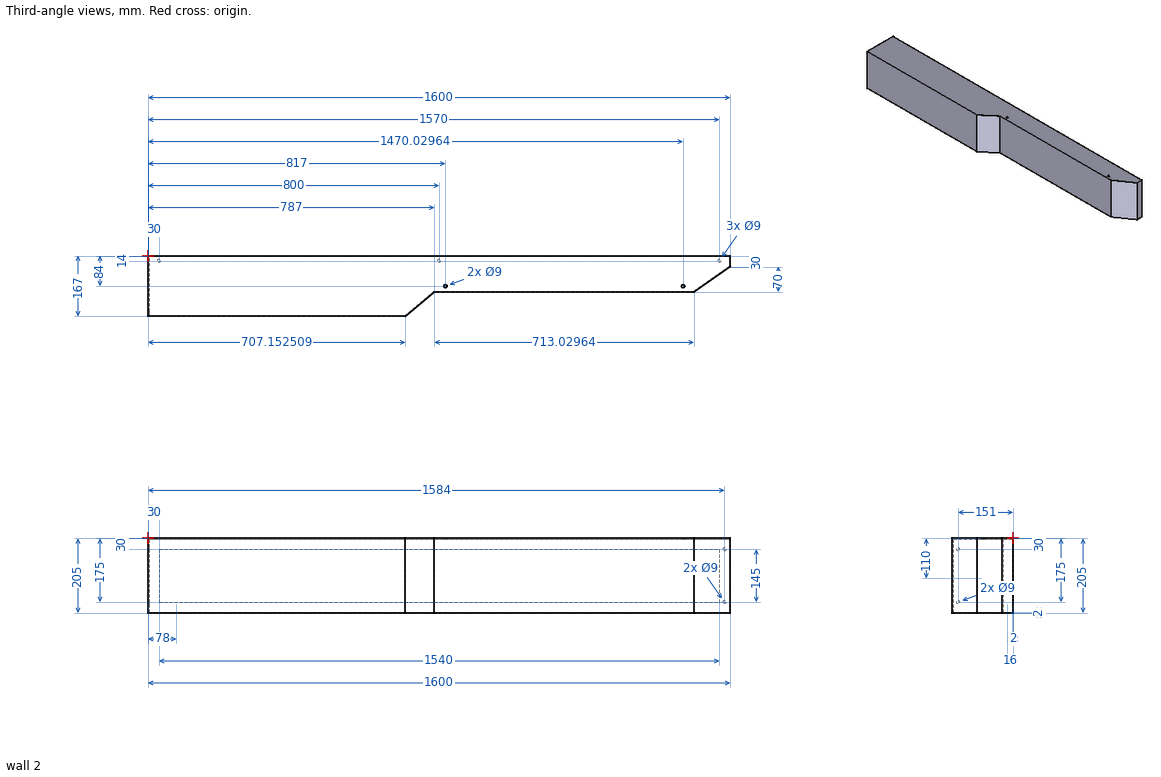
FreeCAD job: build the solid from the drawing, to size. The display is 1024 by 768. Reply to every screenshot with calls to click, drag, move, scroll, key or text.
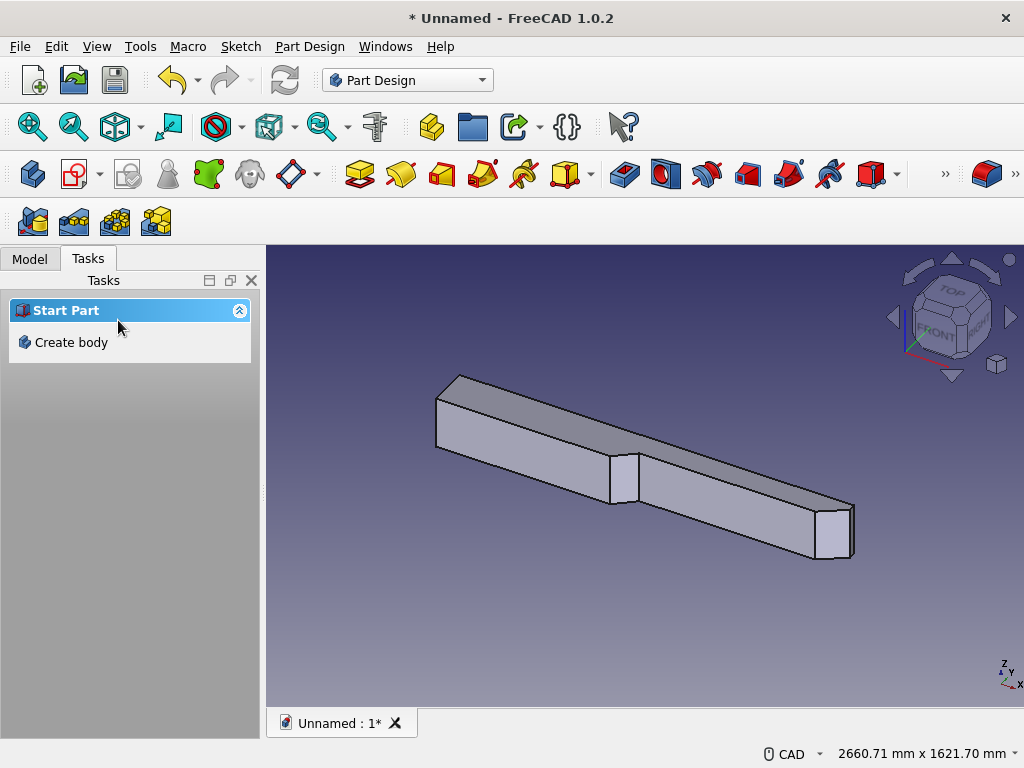
key(0)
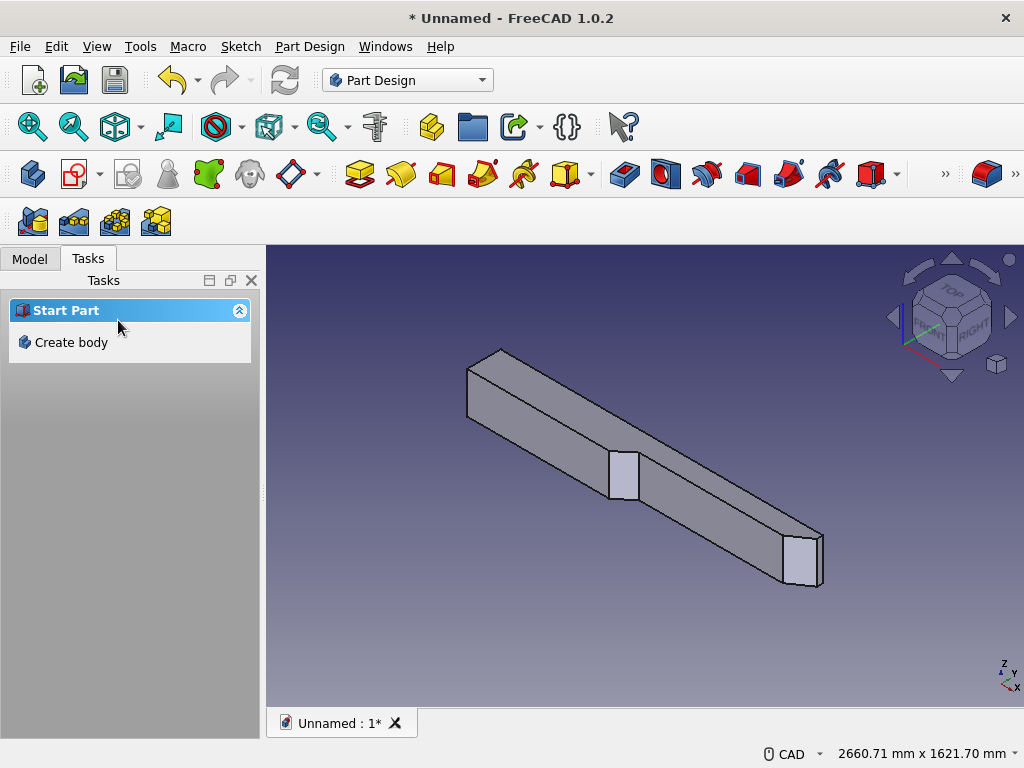
key(2)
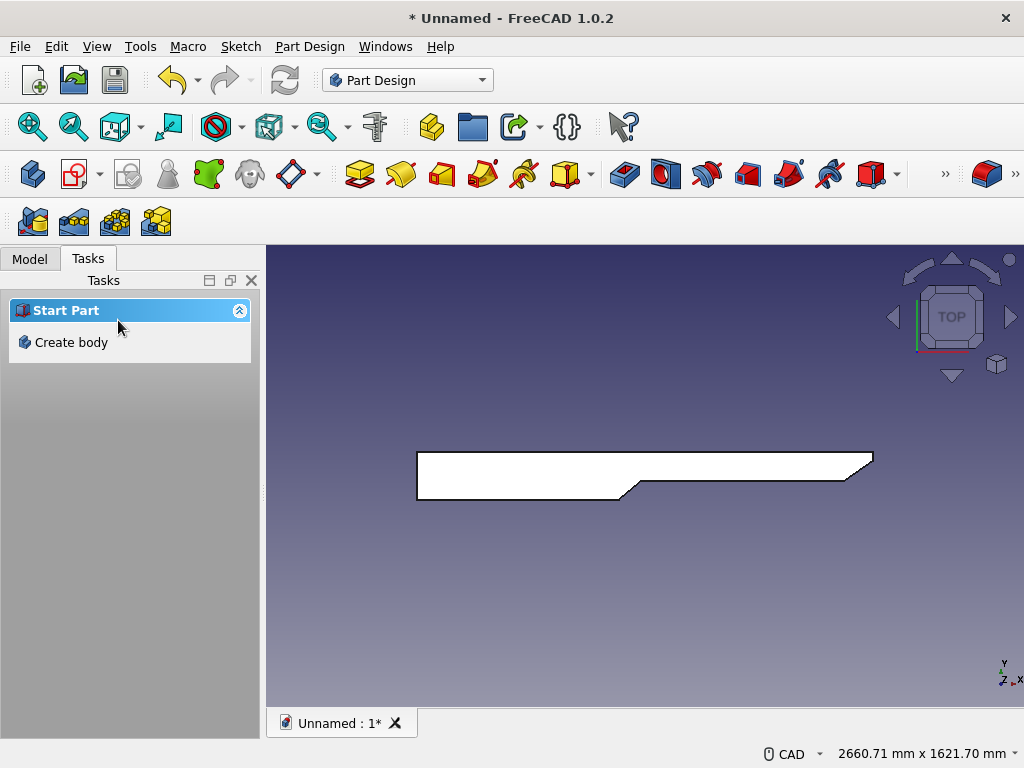
key(1)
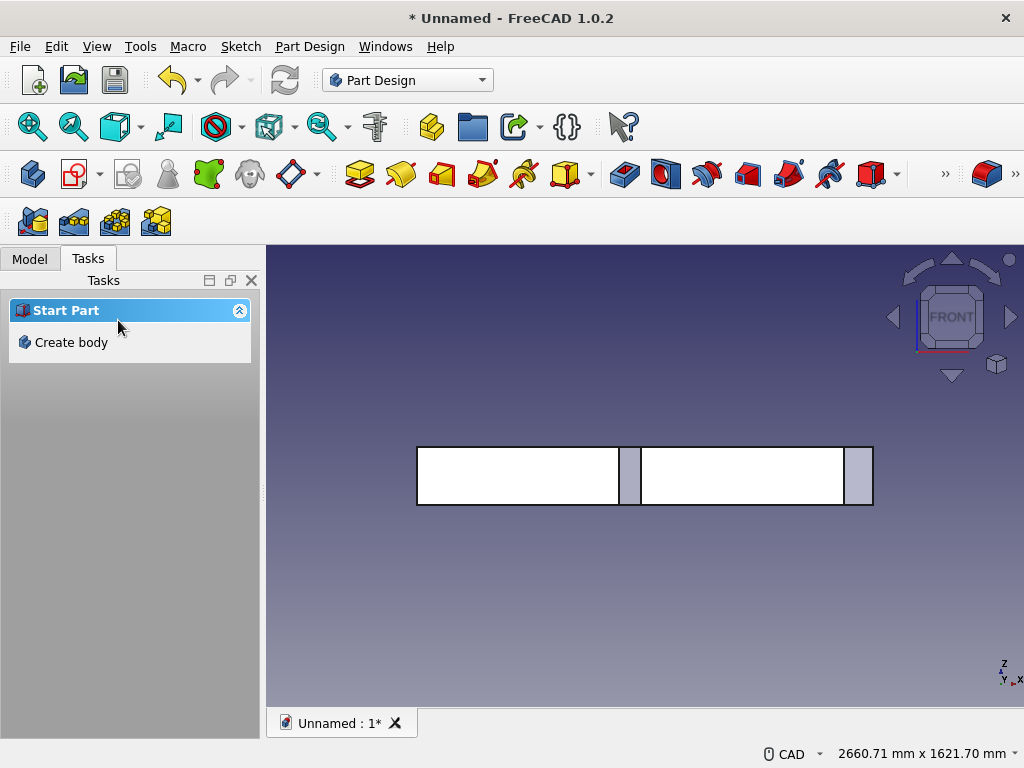
key(3)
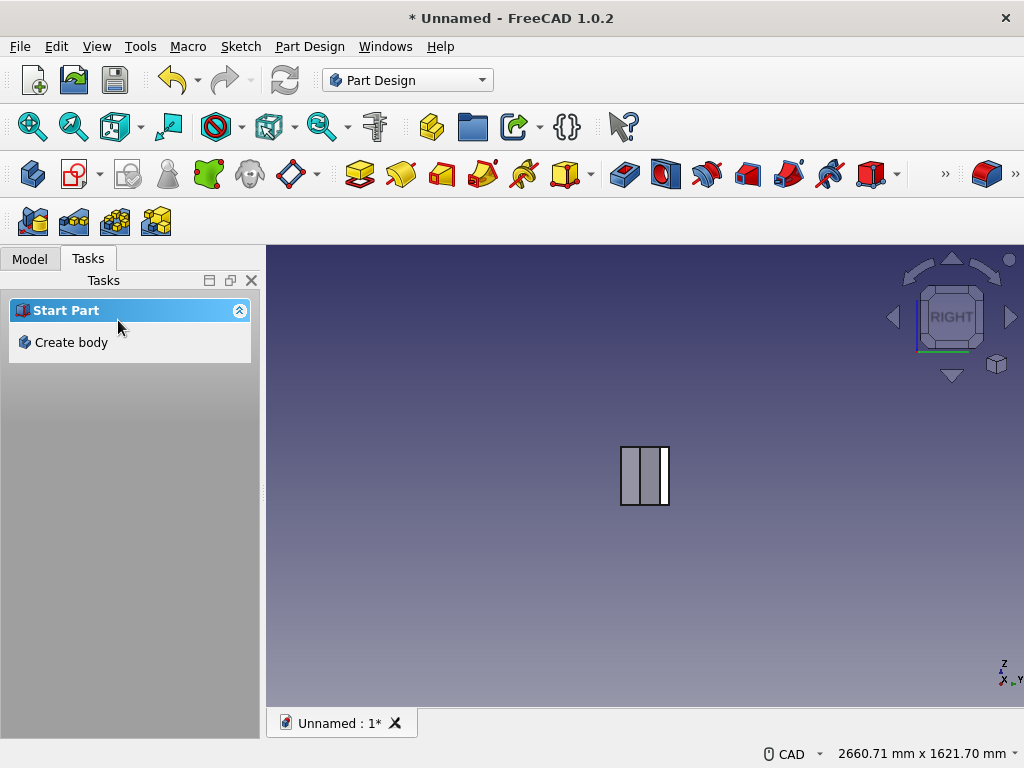
key(v)
key(f)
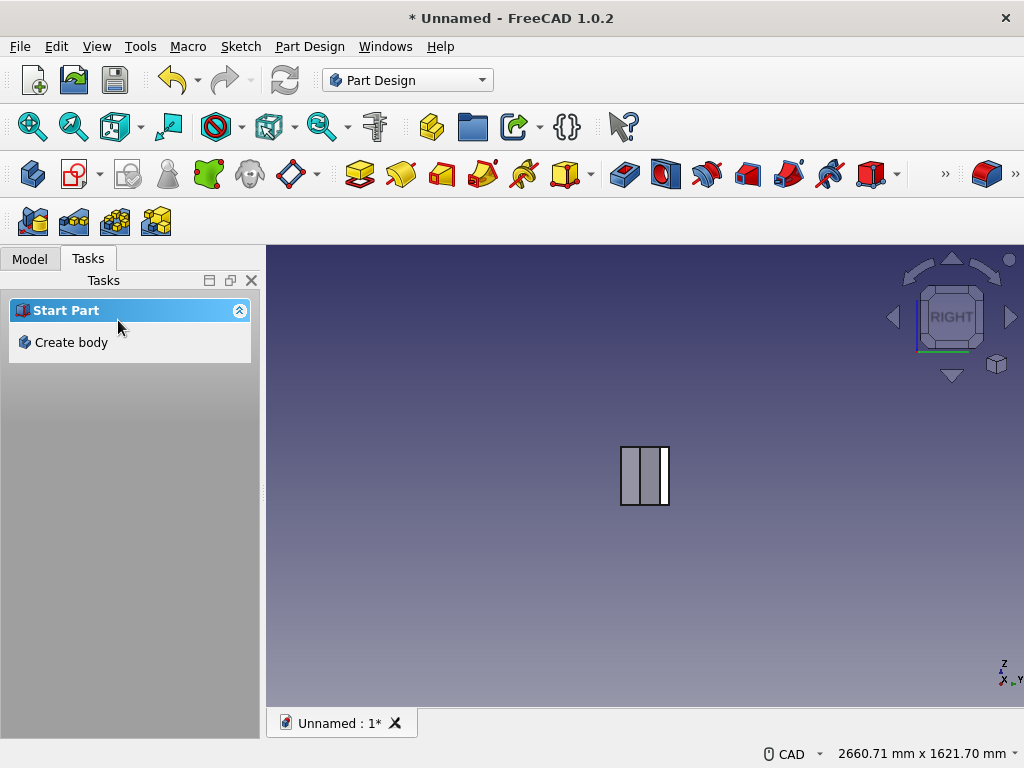
key(5)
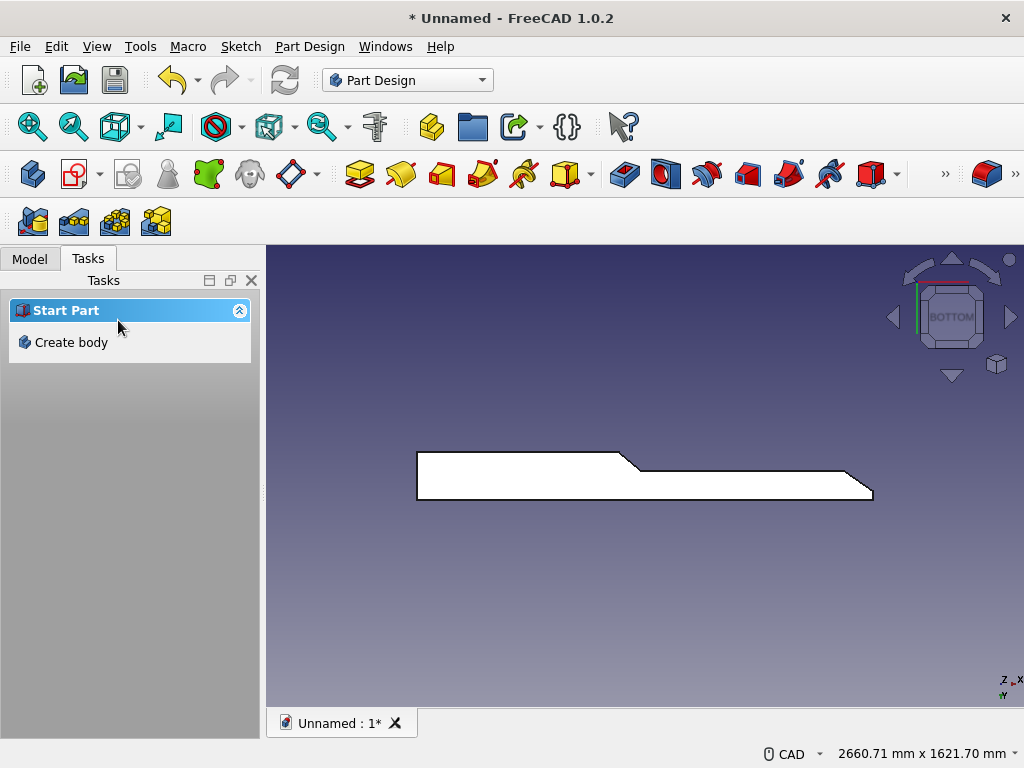
key(4)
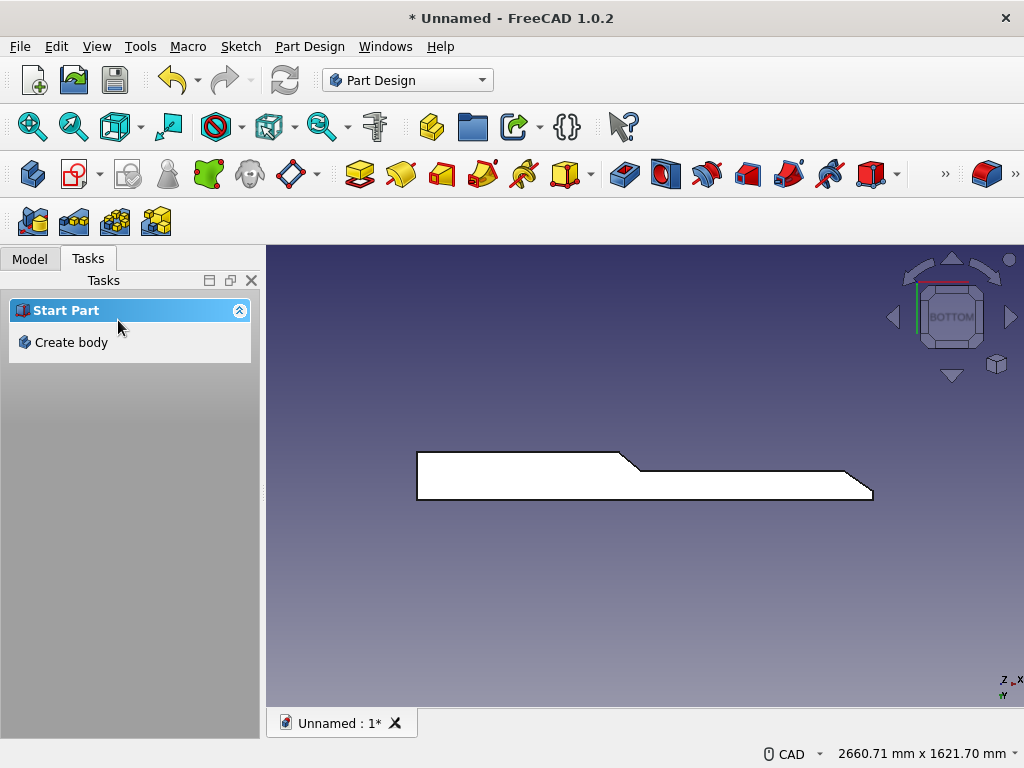
click(450, 475)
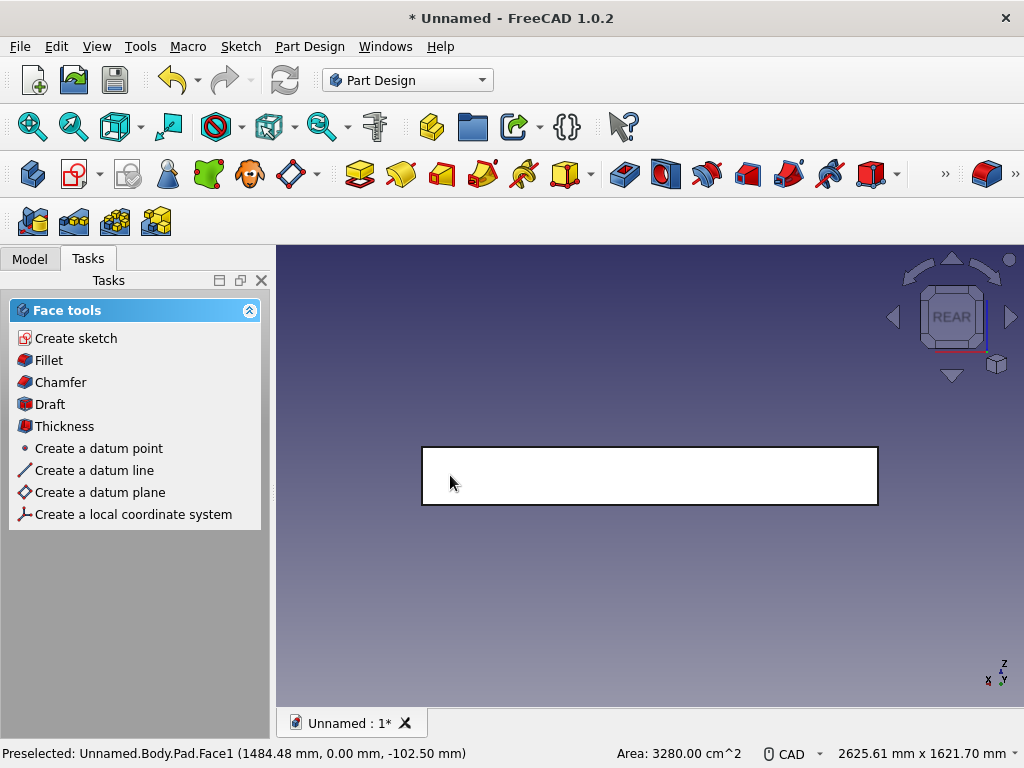
click(135, 426)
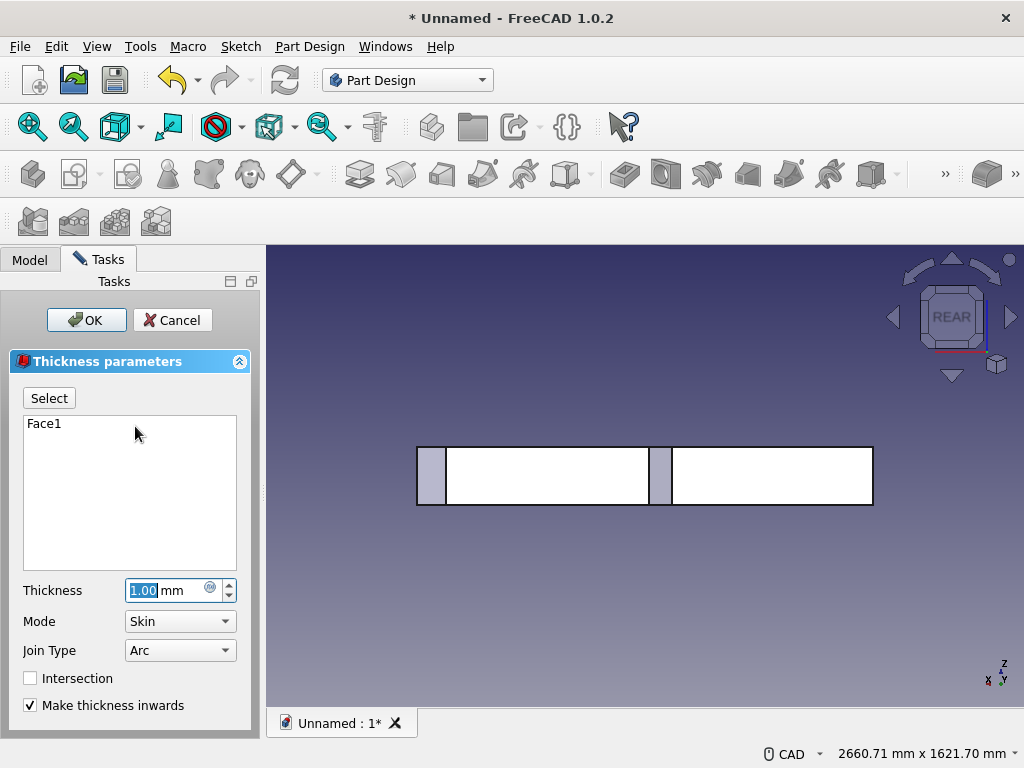
text(2)
key(Tab)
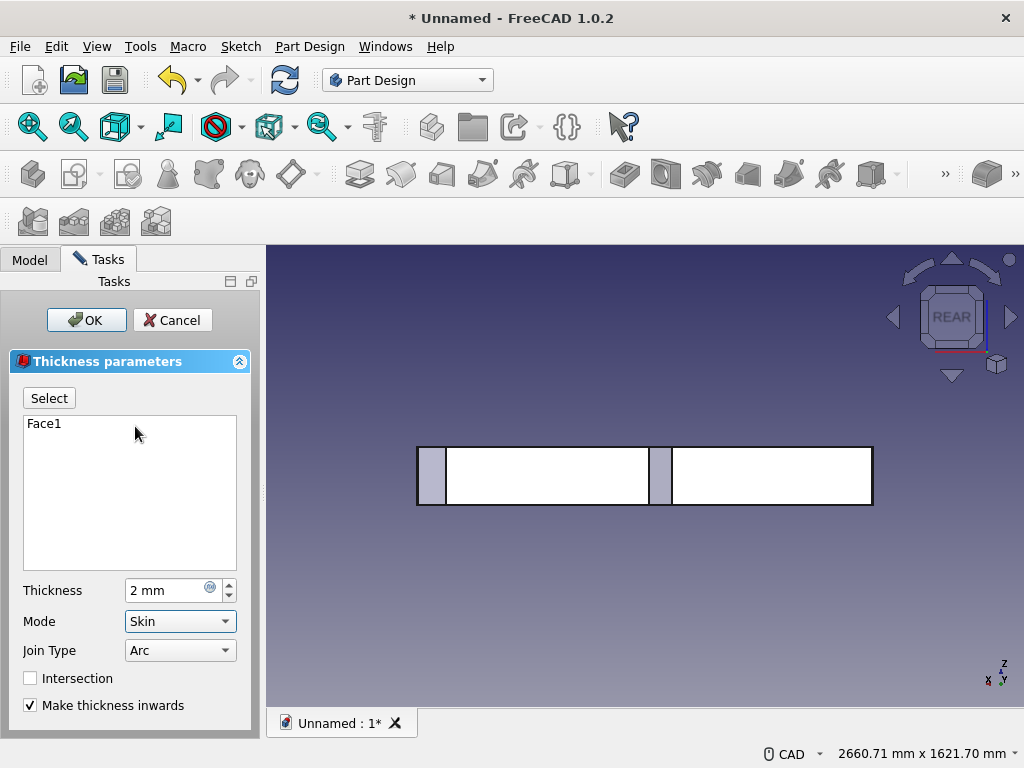
click(181, 650)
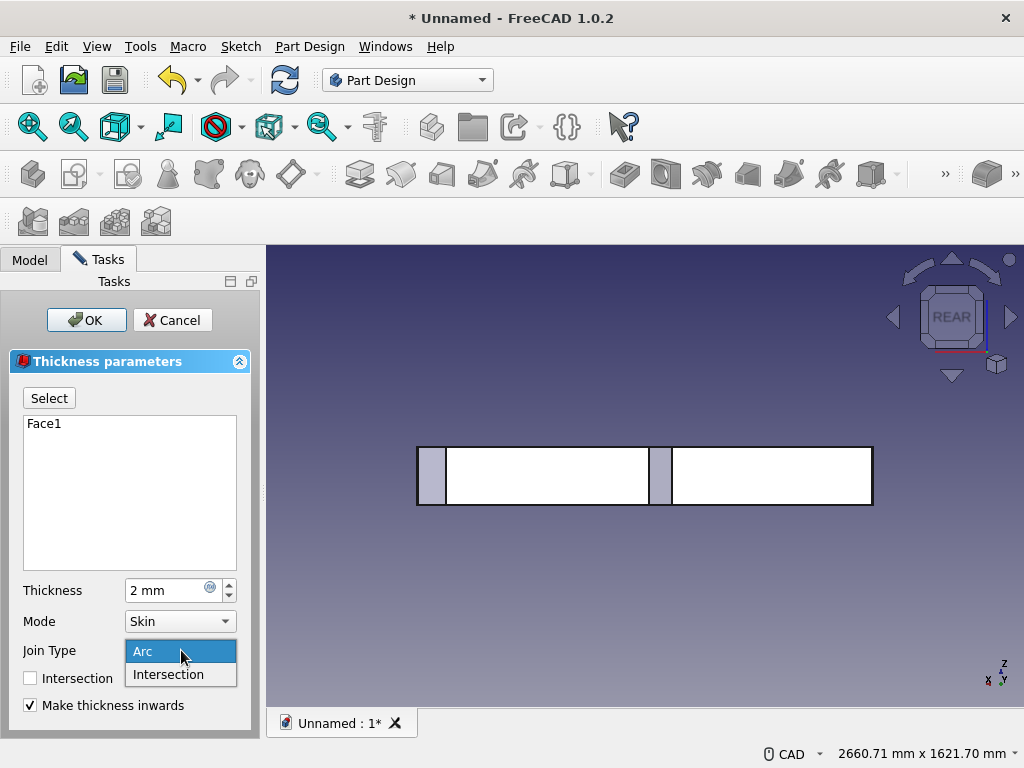
click(179, 674)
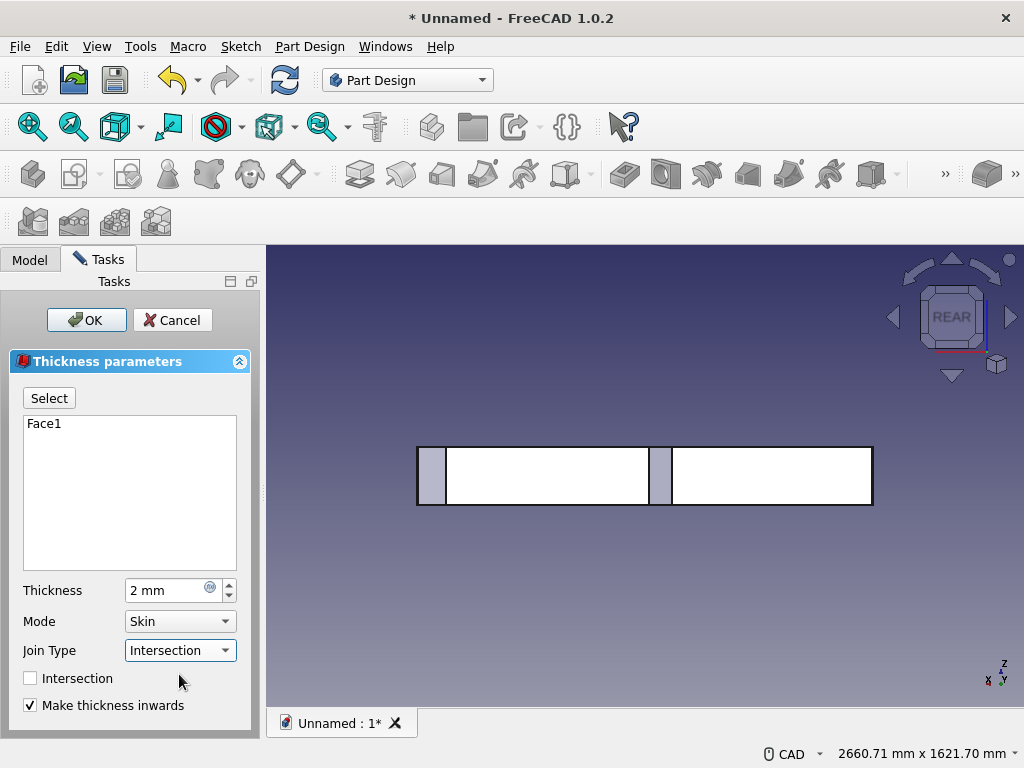
click(87, 320)